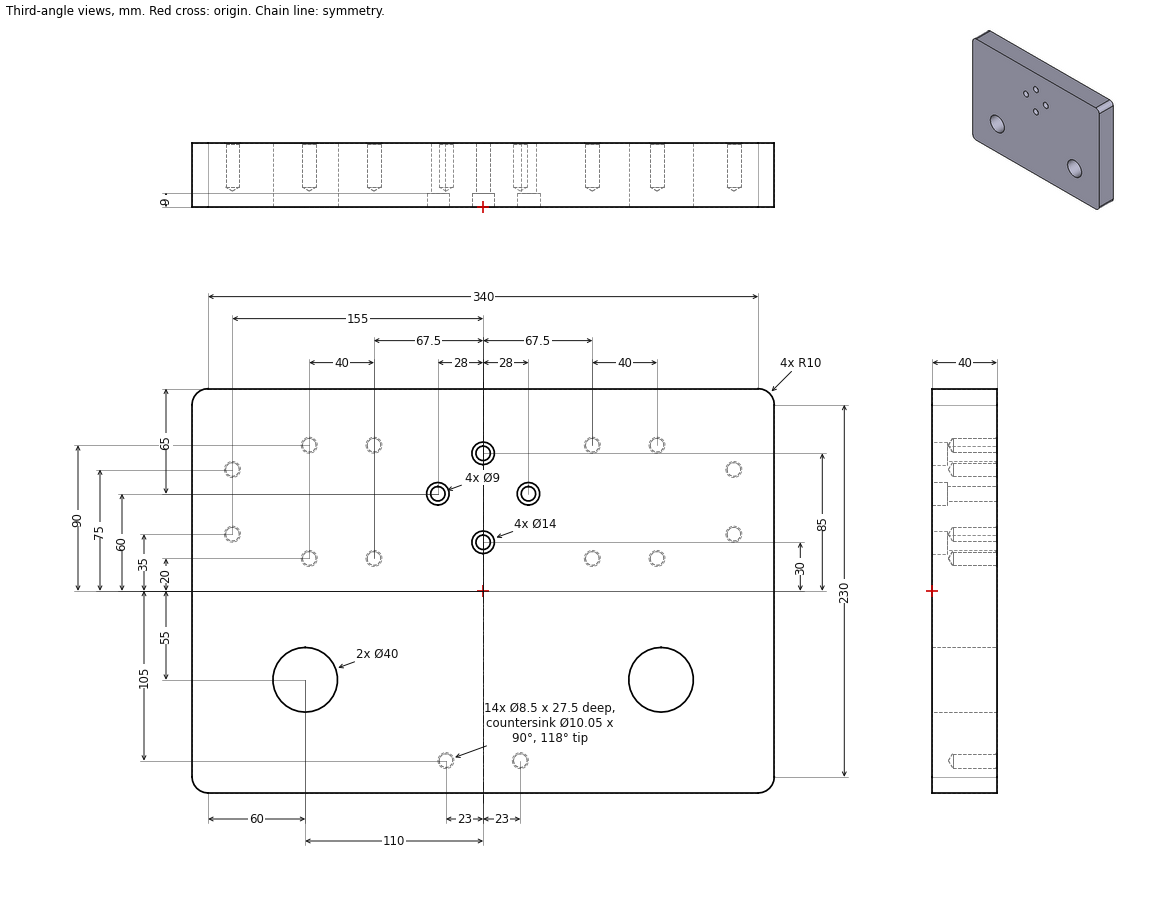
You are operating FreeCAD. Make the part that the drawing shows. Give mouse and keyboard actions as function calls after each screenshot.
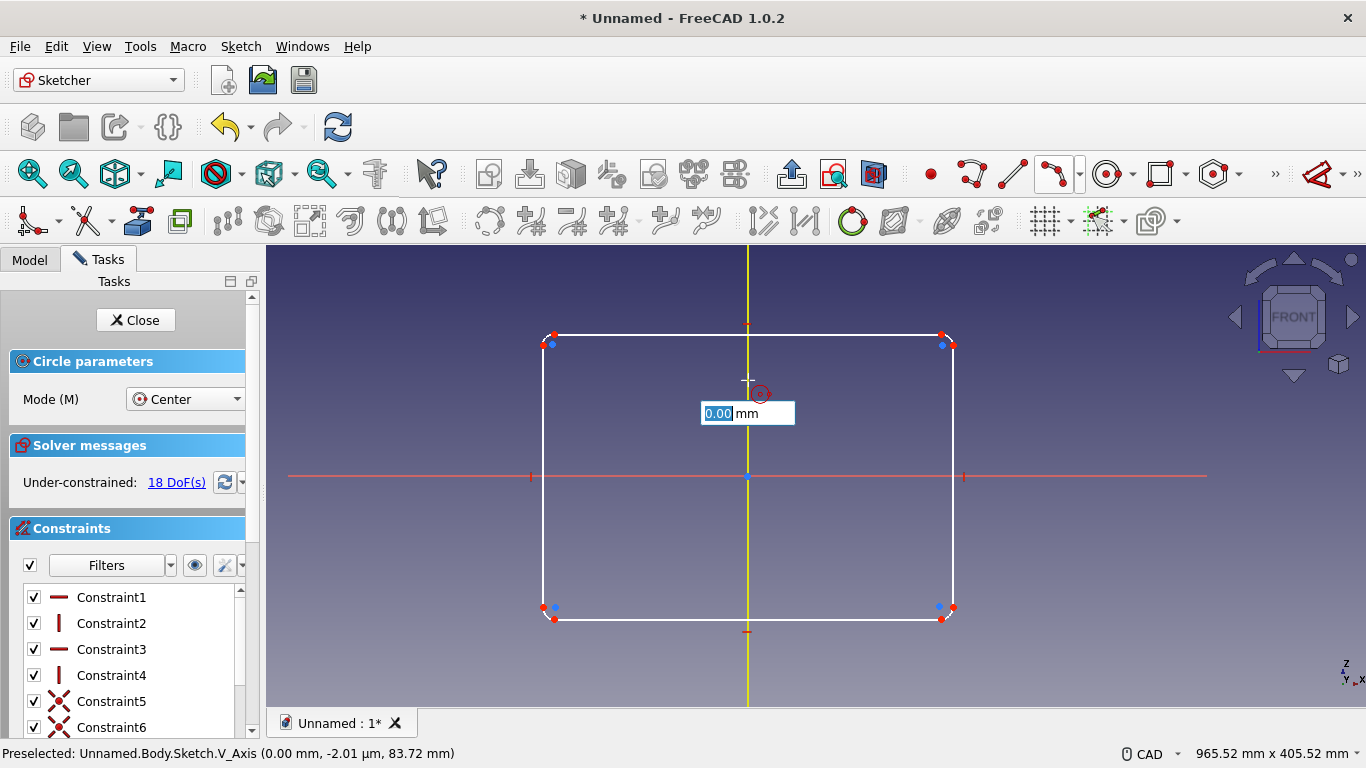
scroll(753, 378, up, 6)
move(751, 377)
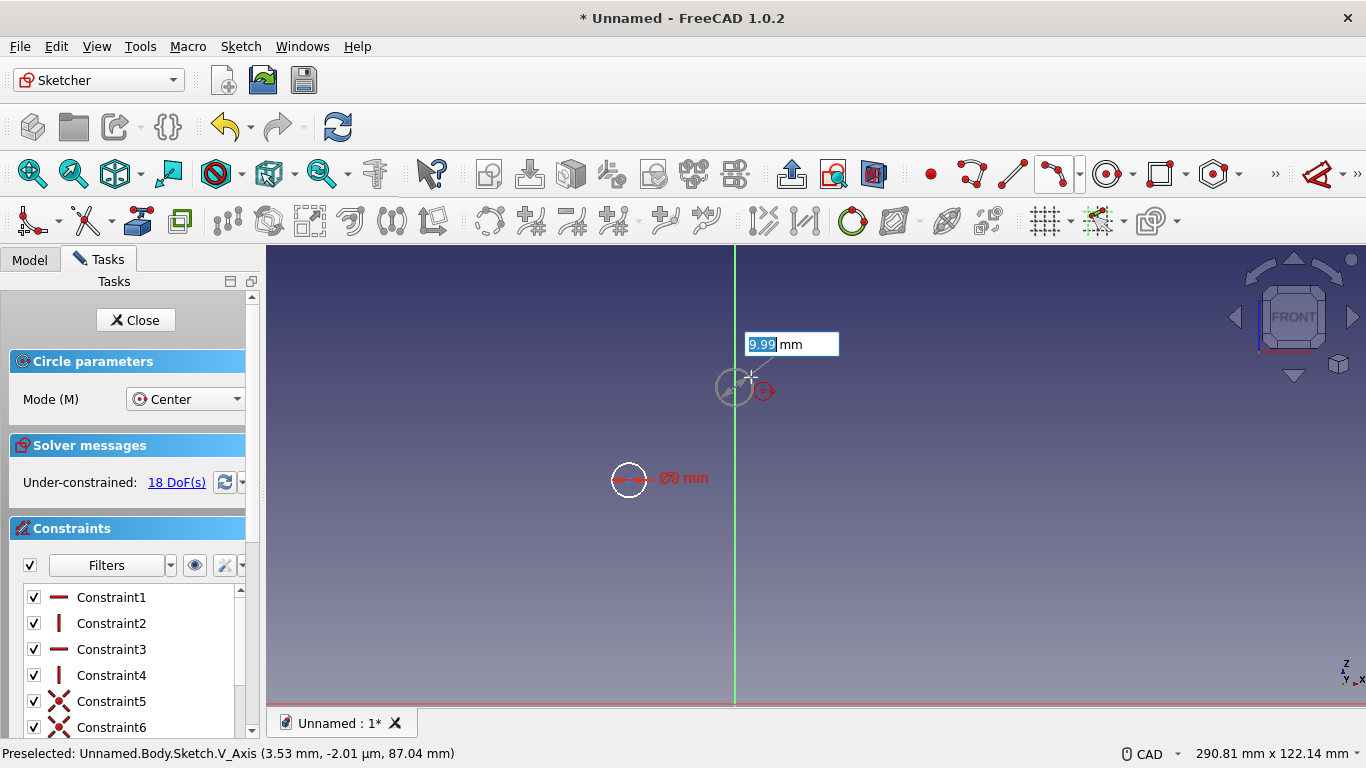
text(9)
key(Return)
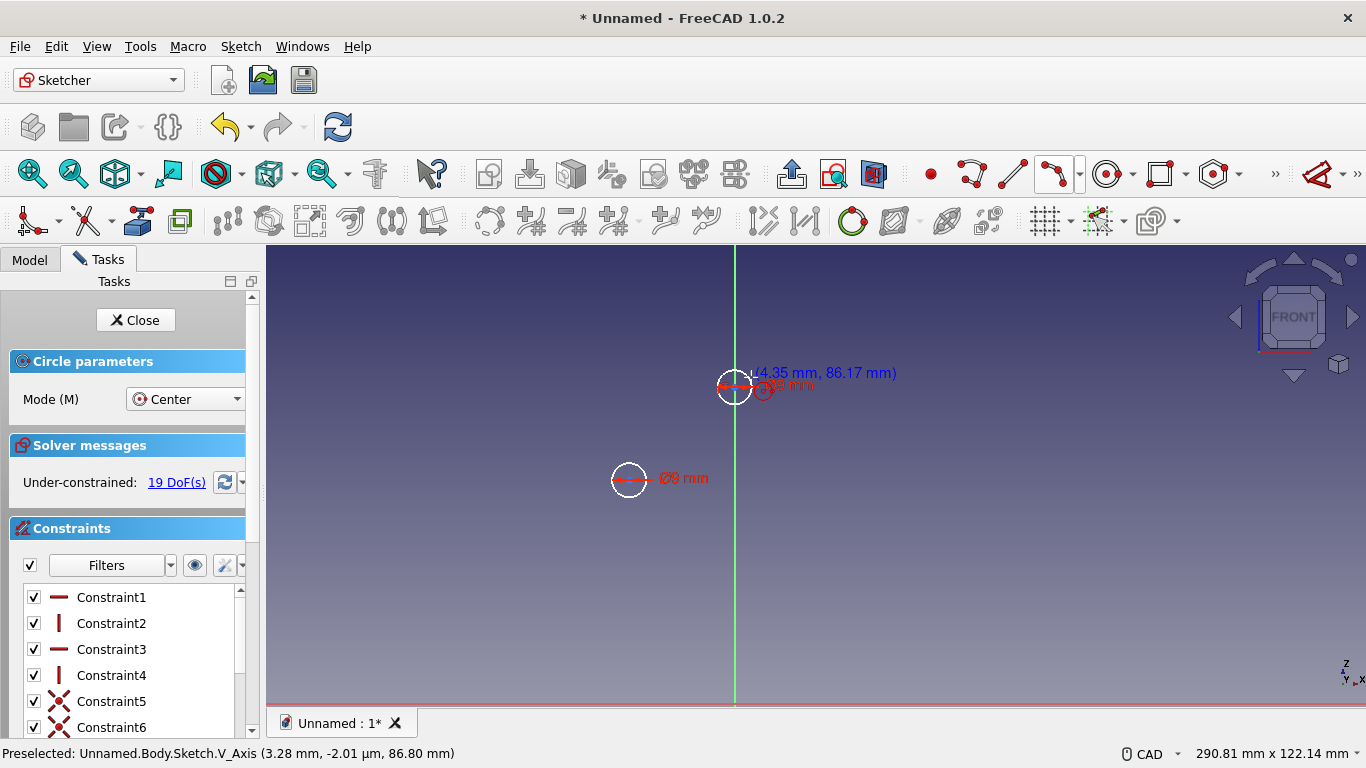
scroll(840, 477, up, 2)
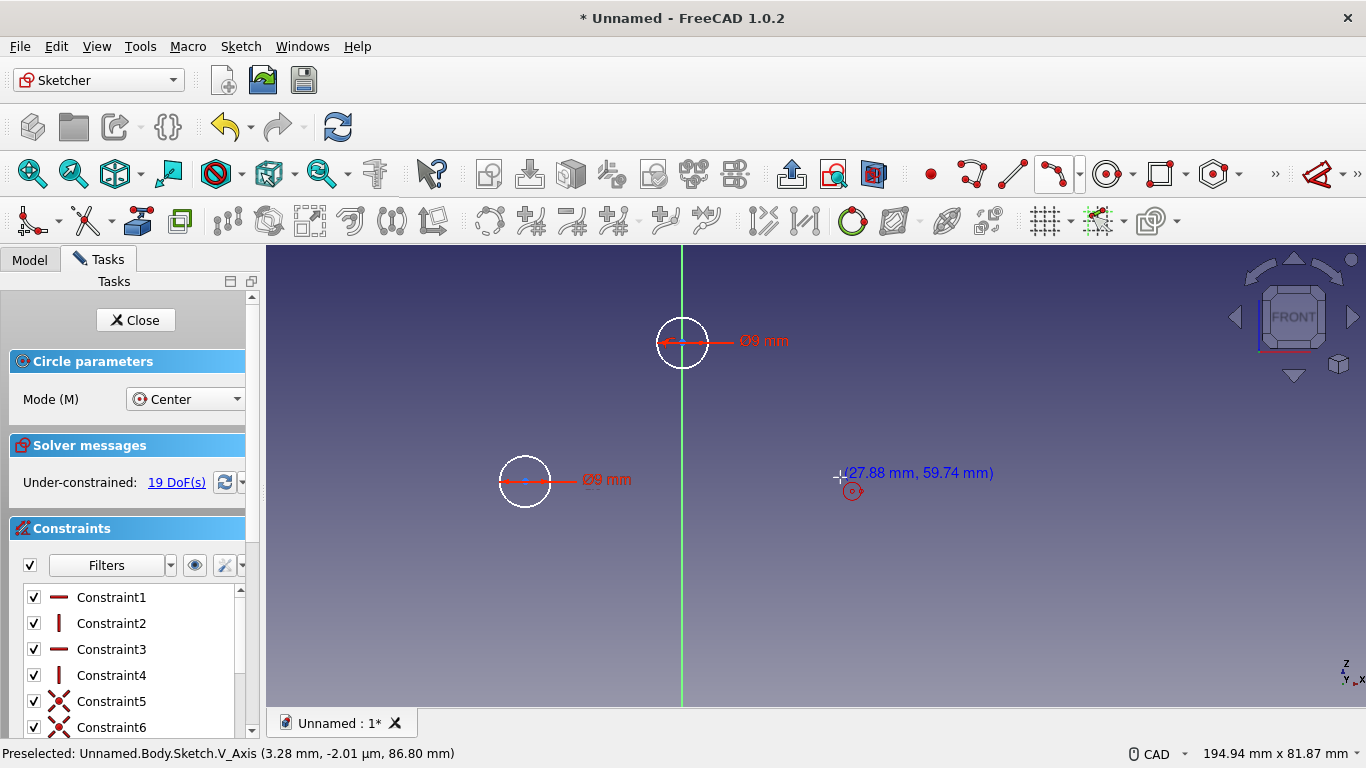
scroll(764, 390, down, 8)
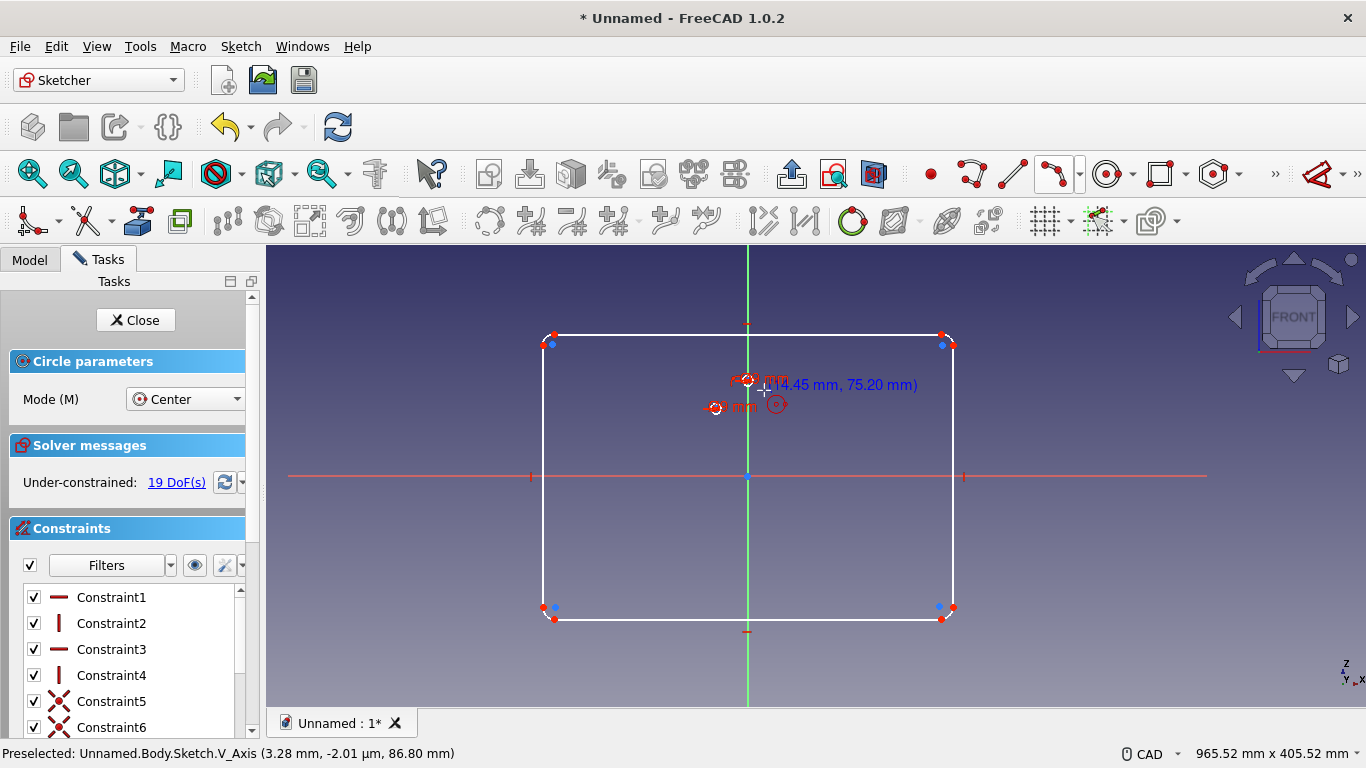
click(780, 408)
move(783, 404)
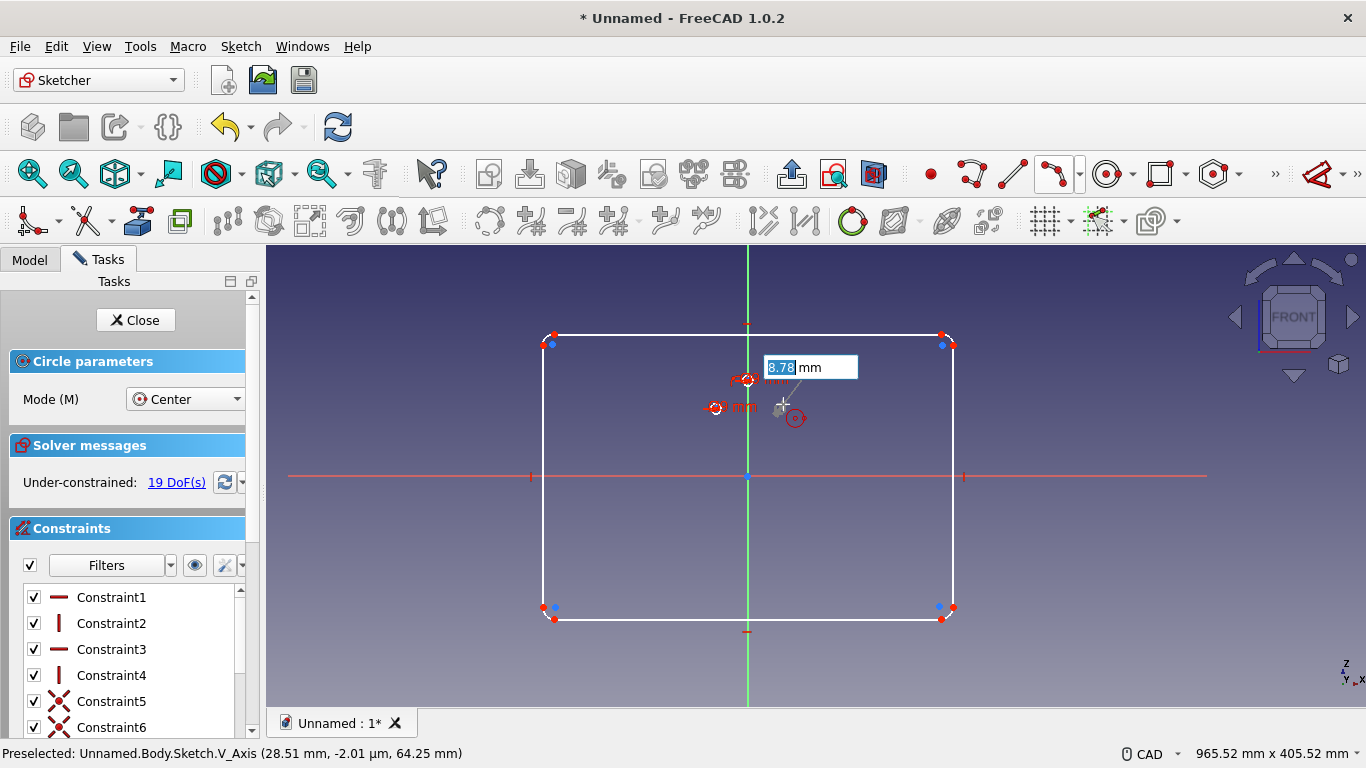
text(9)
key(Return)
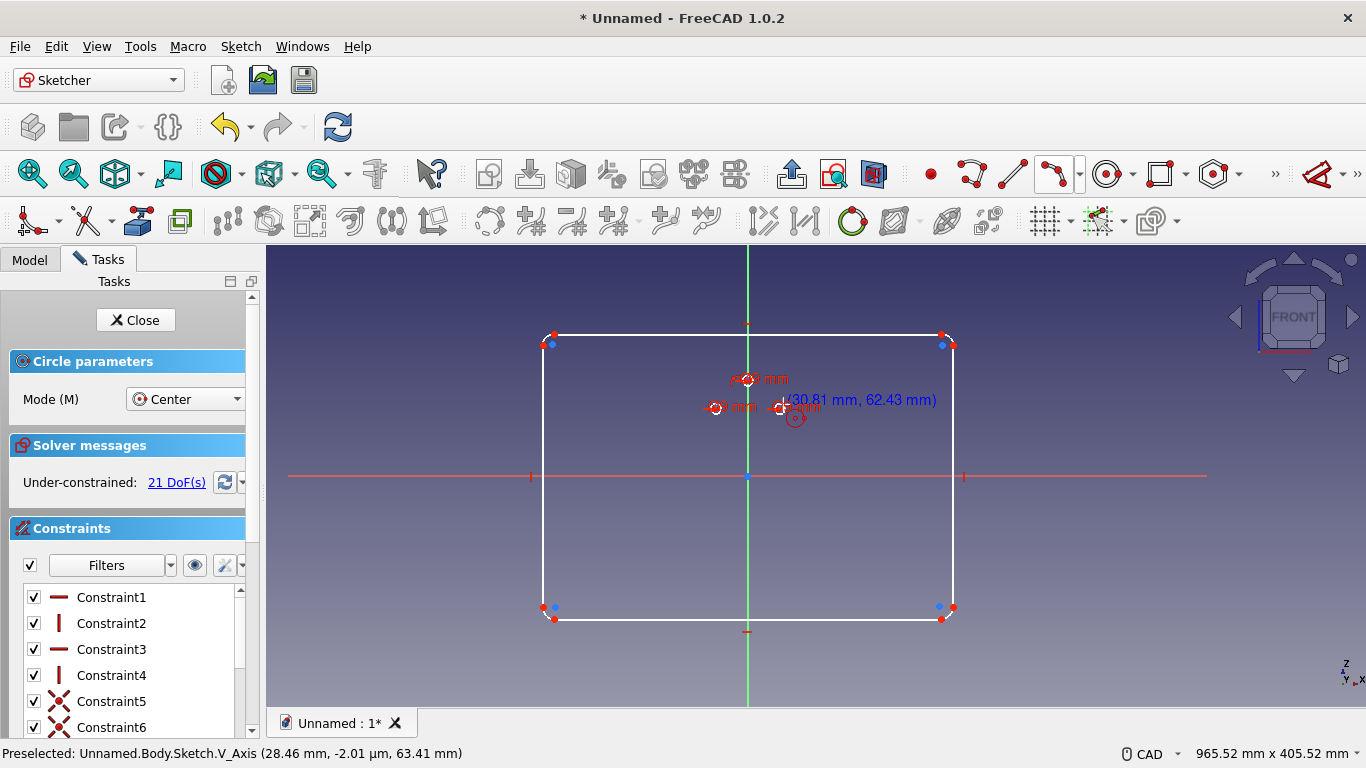
scroll(748, 442, up, 8)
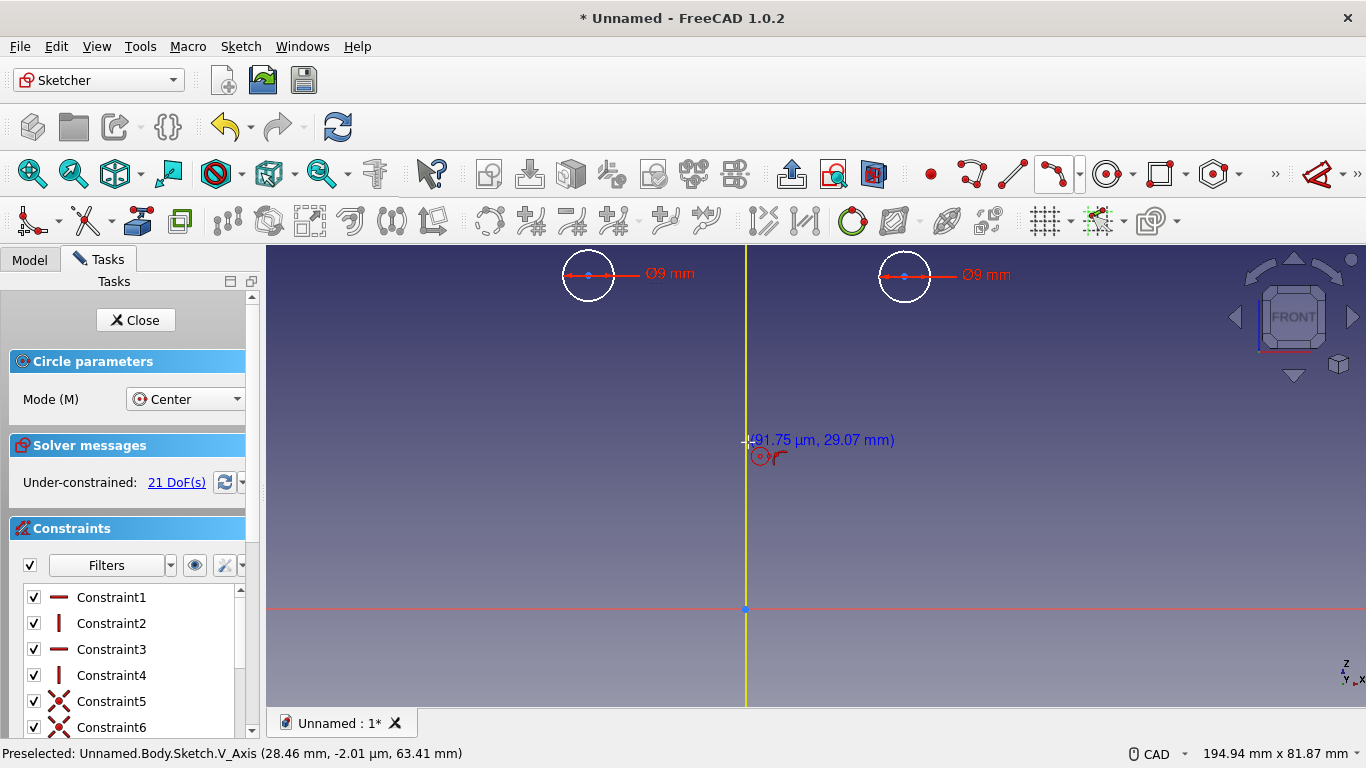
scroll(748, 442, down, 8)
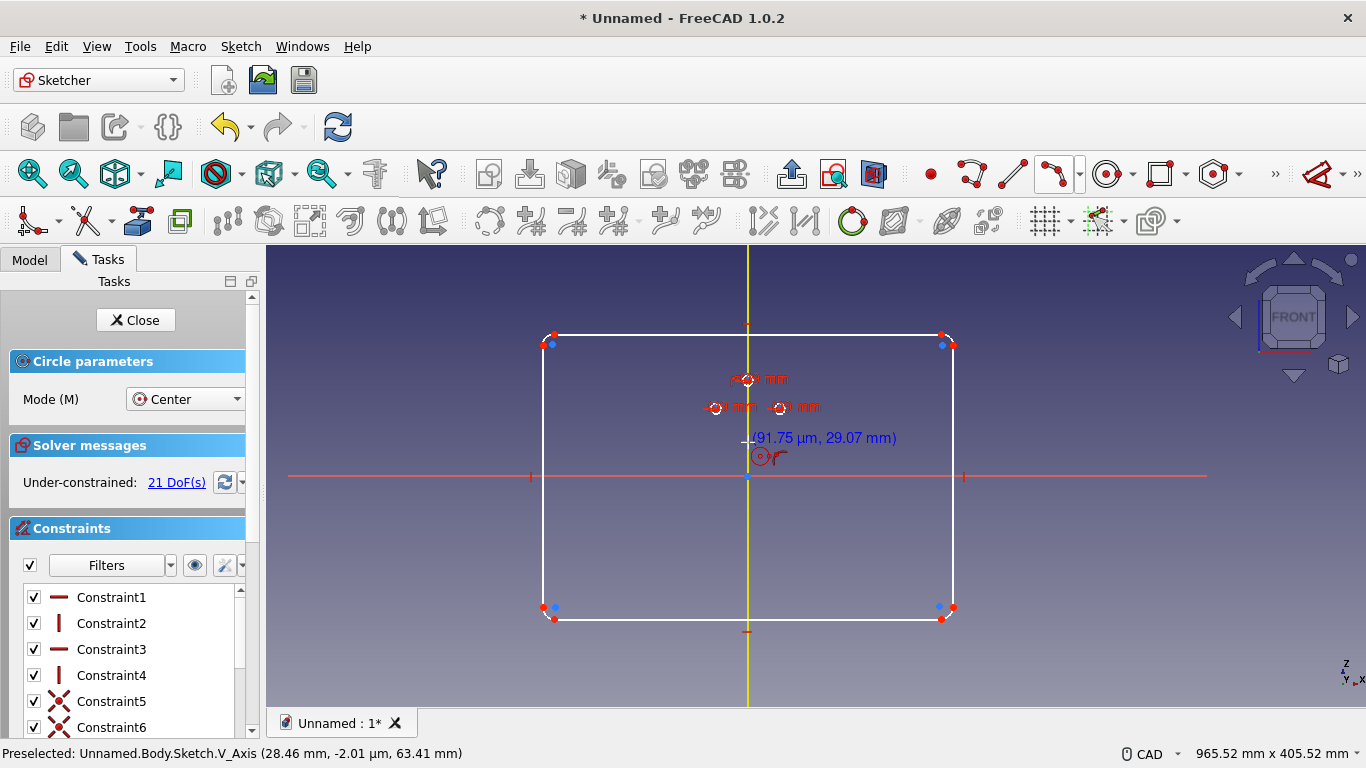
click(748, 442)